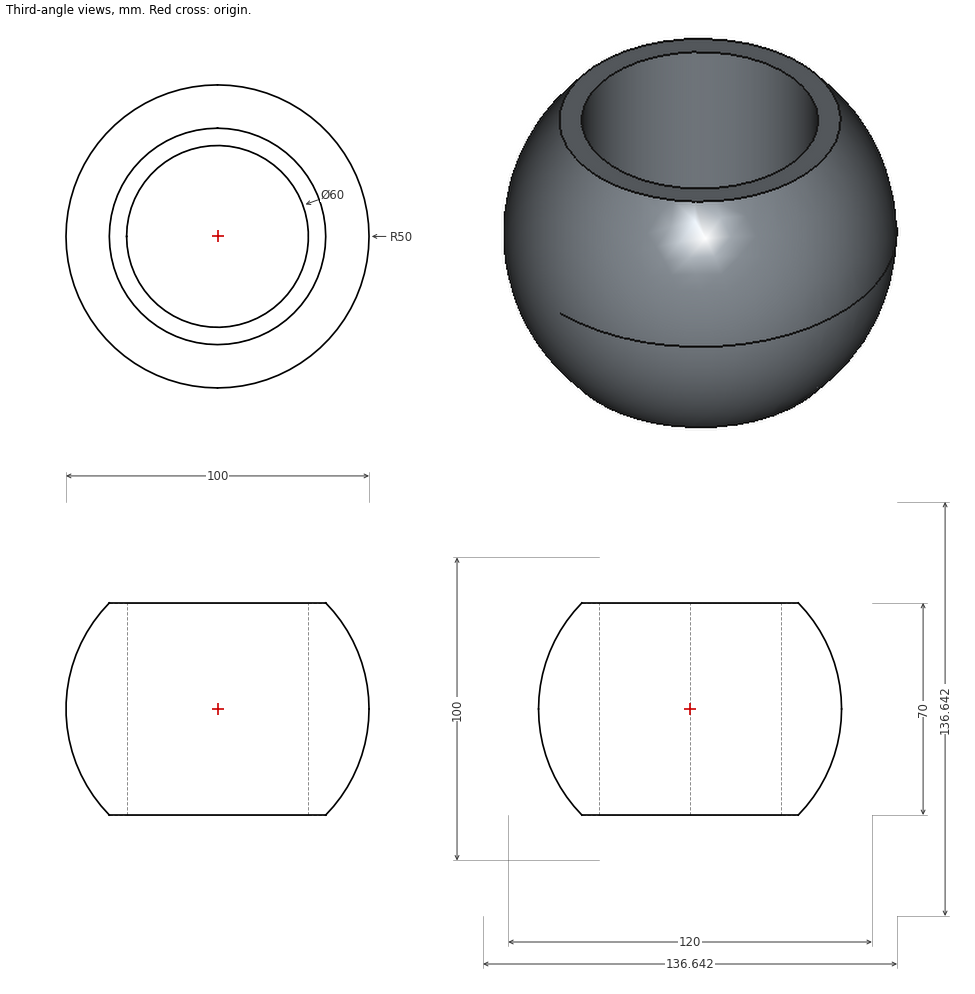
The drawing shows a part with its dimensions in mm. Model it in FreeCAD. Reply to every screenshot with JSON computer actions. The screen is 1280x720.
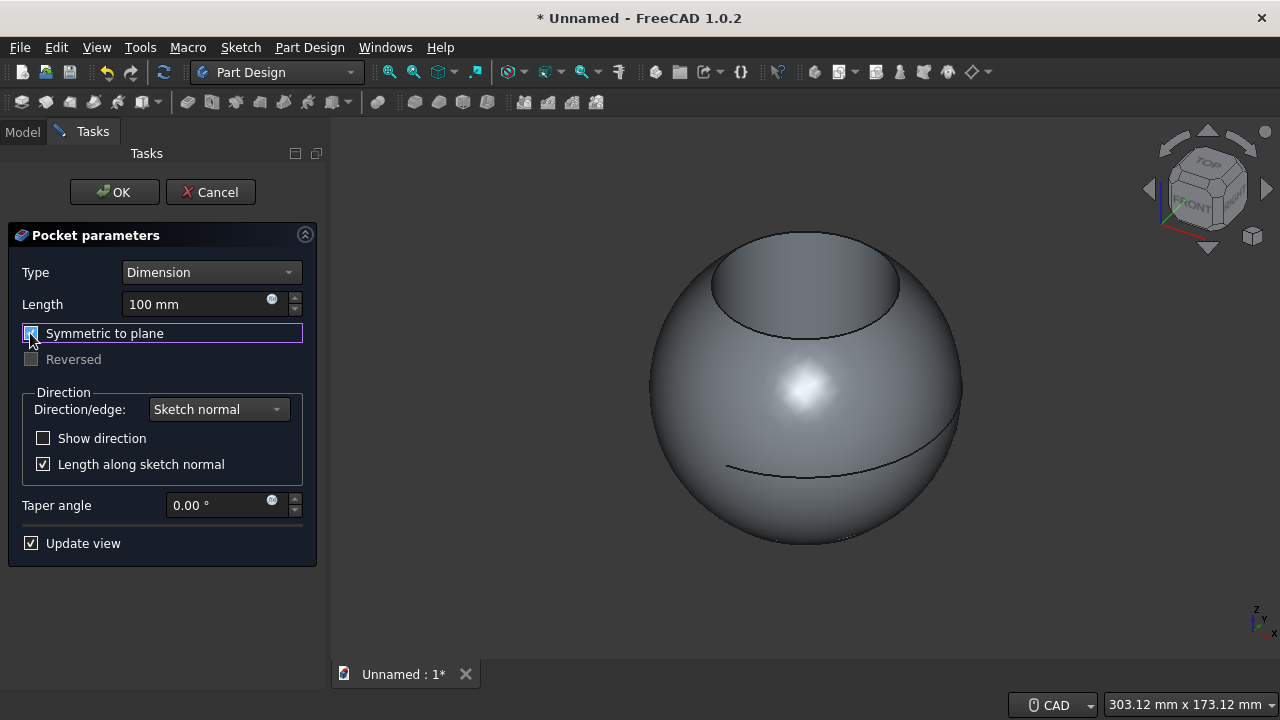
{"action": "left_click", "coordinate": [115, 192]}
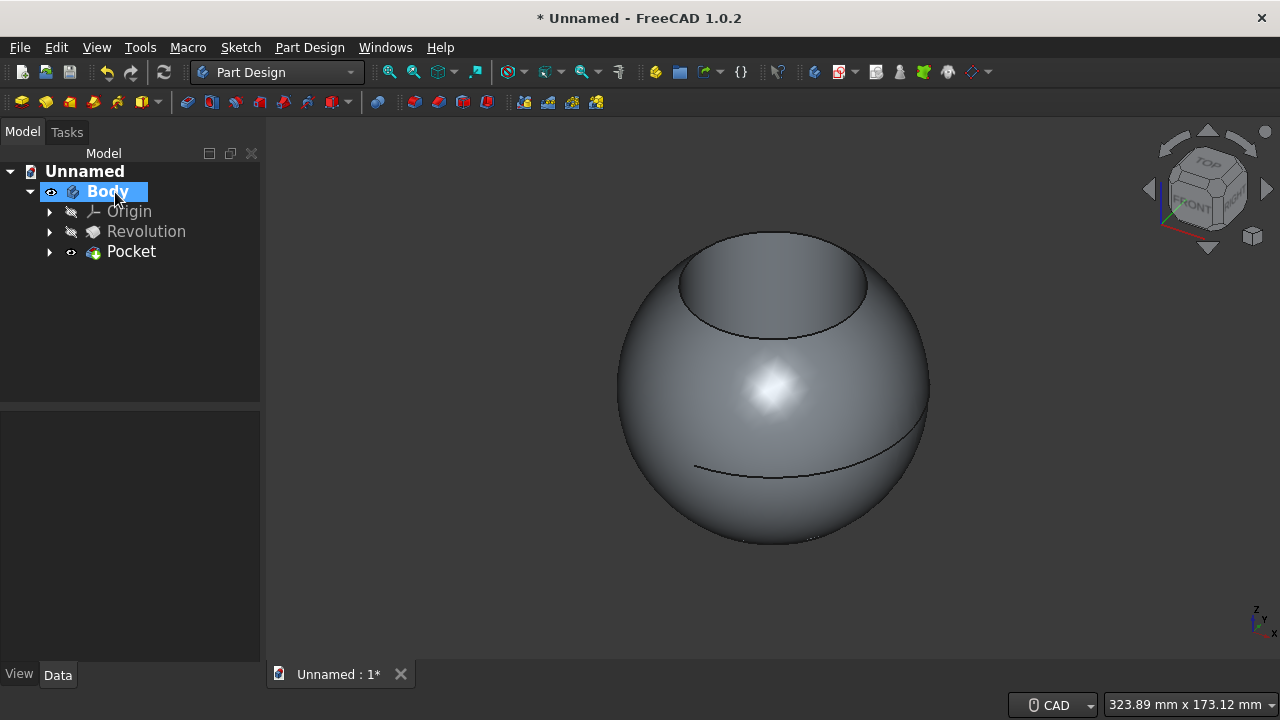
{"action": "left_click", "coordinate": [840, 72]}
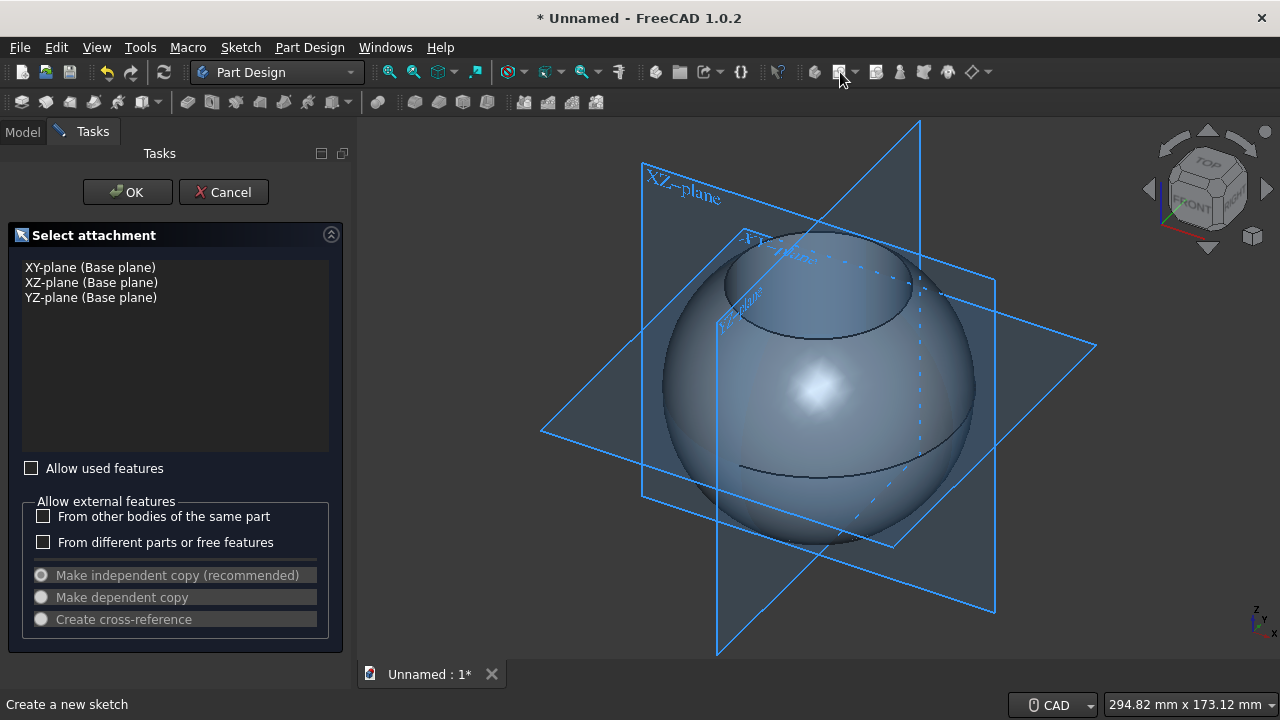
{"action": "left_click", "coordinate": [82, 298]}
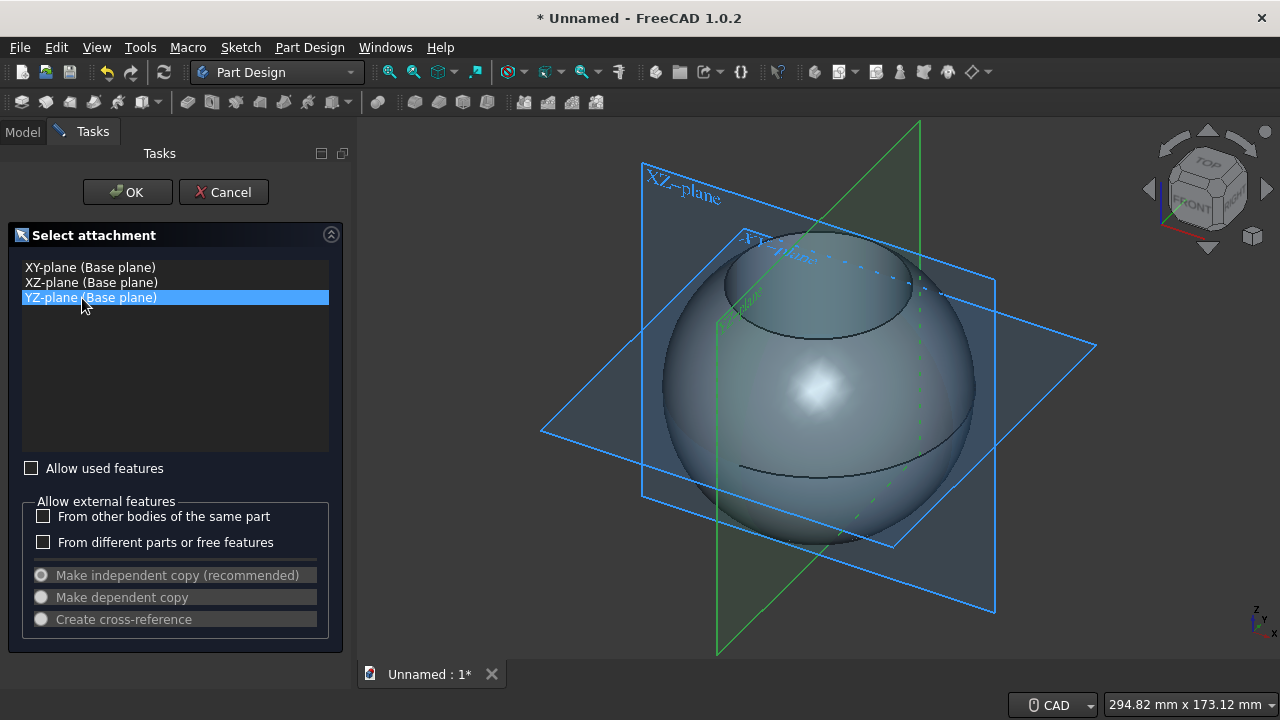
{"action": "left_click", "coordinate": [128, 192]}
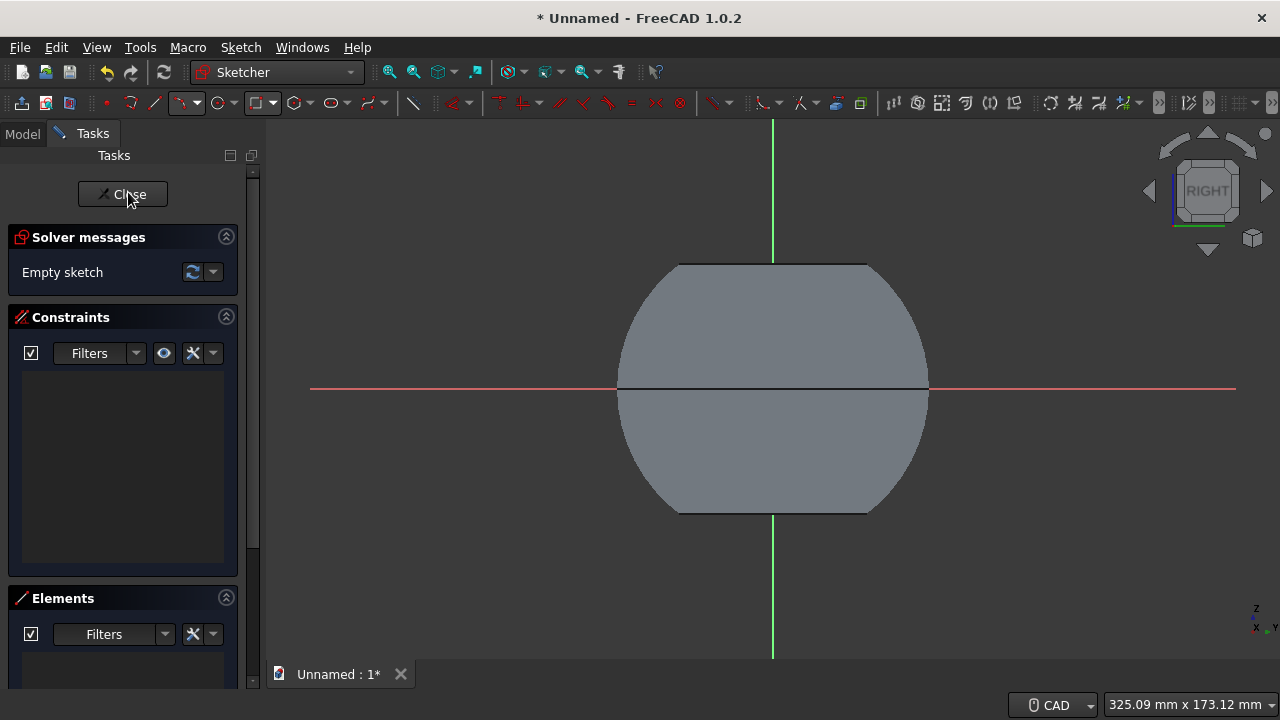
{"action": "left_click", "coordinate": [70, 104]}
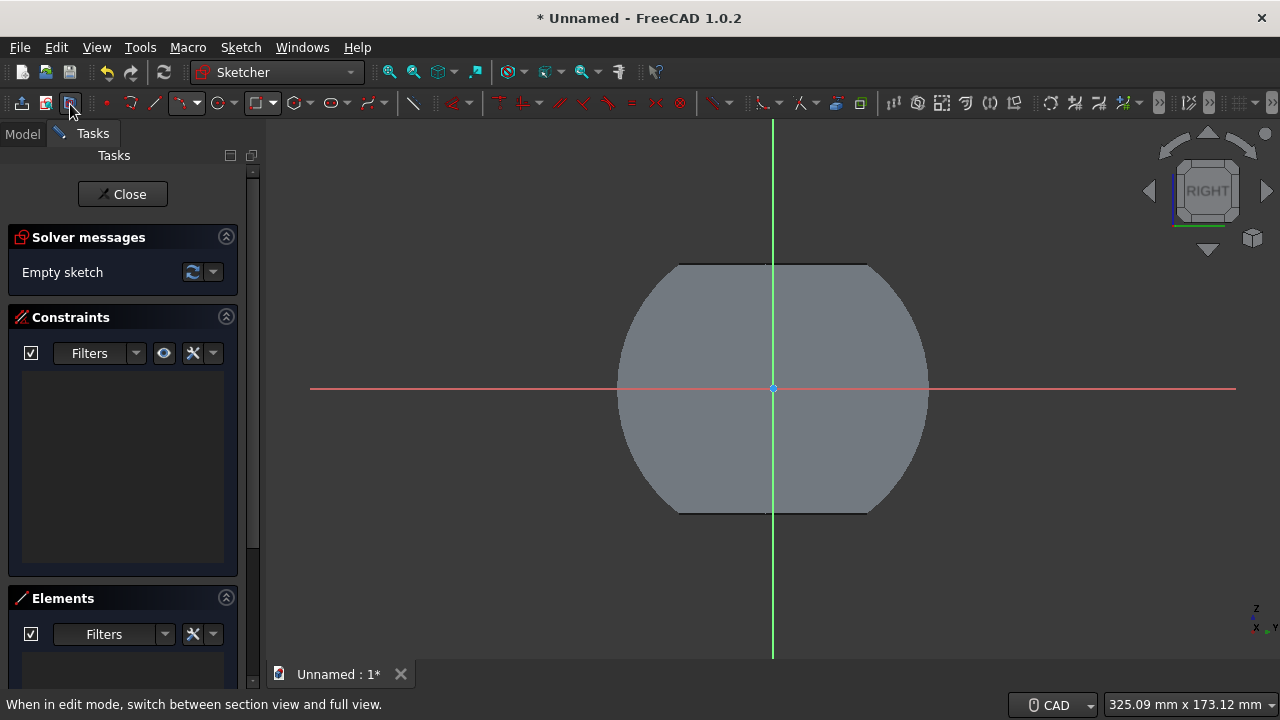
{"action": "key", "text": "g v"}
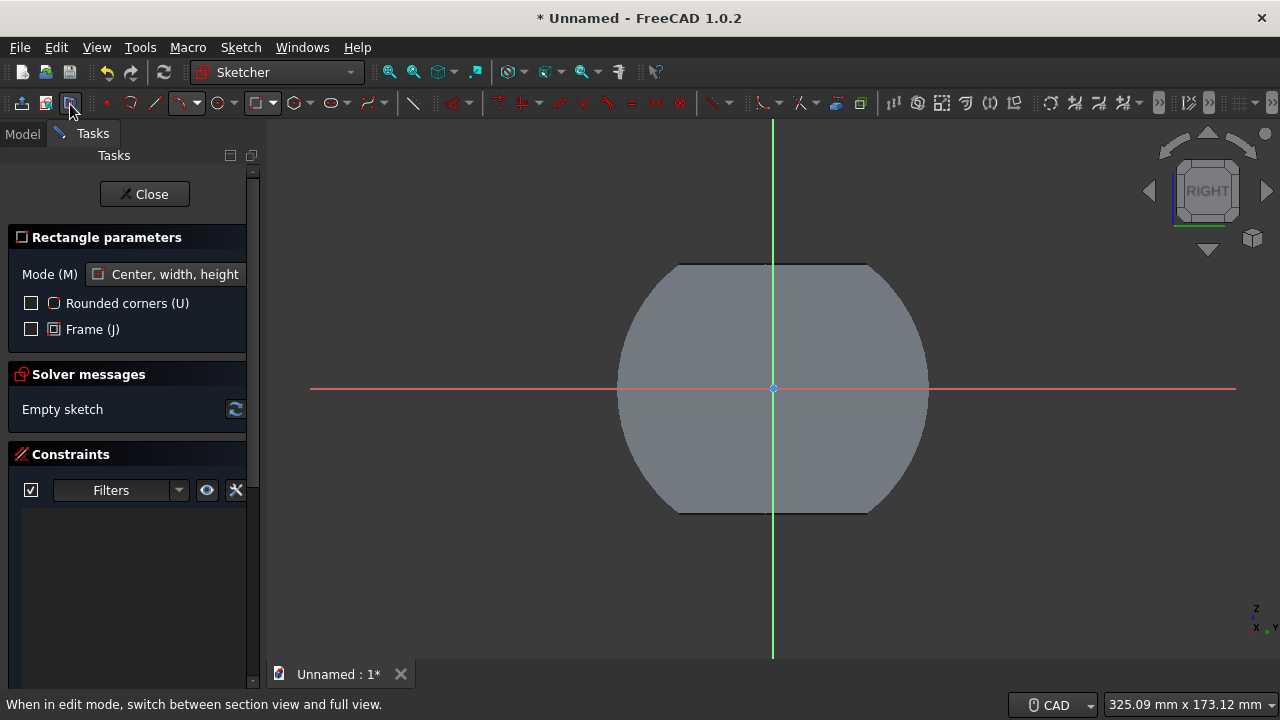
{"action": "left_click", "coordinate": [773, 389]}
{"action": "left_click", "coordinate": [986, 176]}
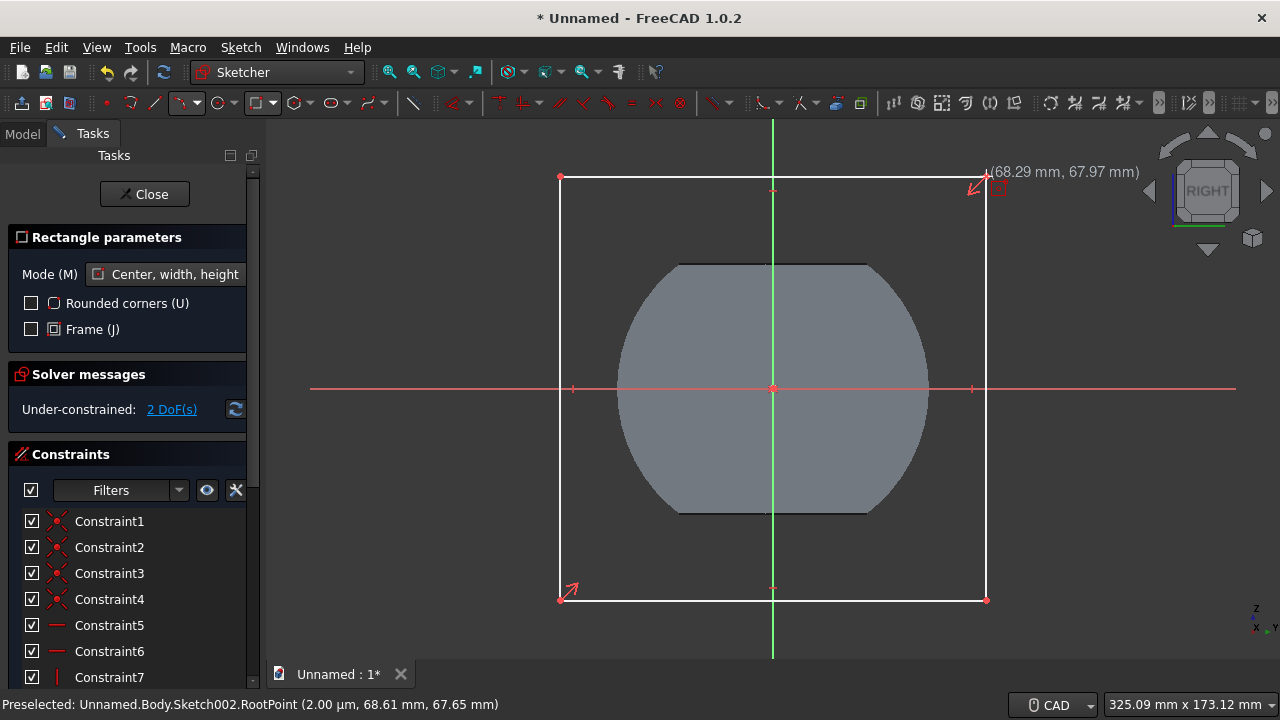
{"action": "left_click", "coordinate": [773, 389]}
{"action": "left_click", "coordinate": [960, 280]}
{"action": "key", "text": "Escape"}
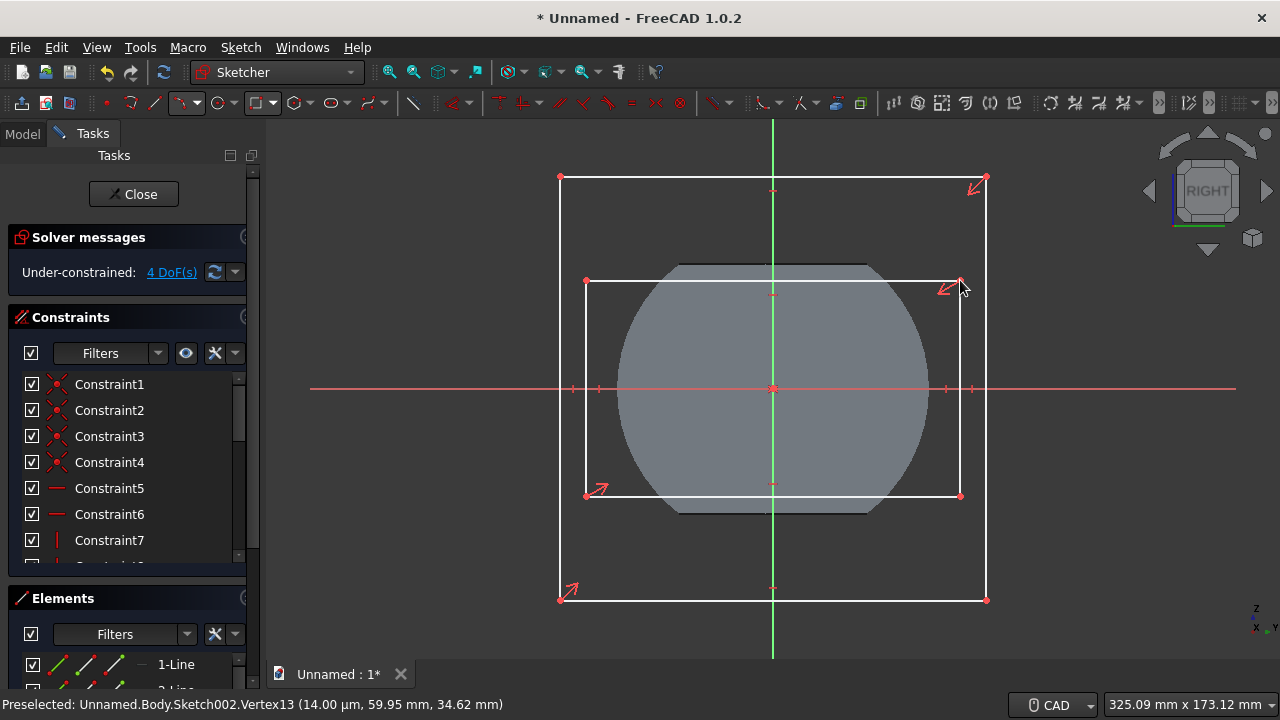
{"action": "left_click", "coordinate": [452, 104]}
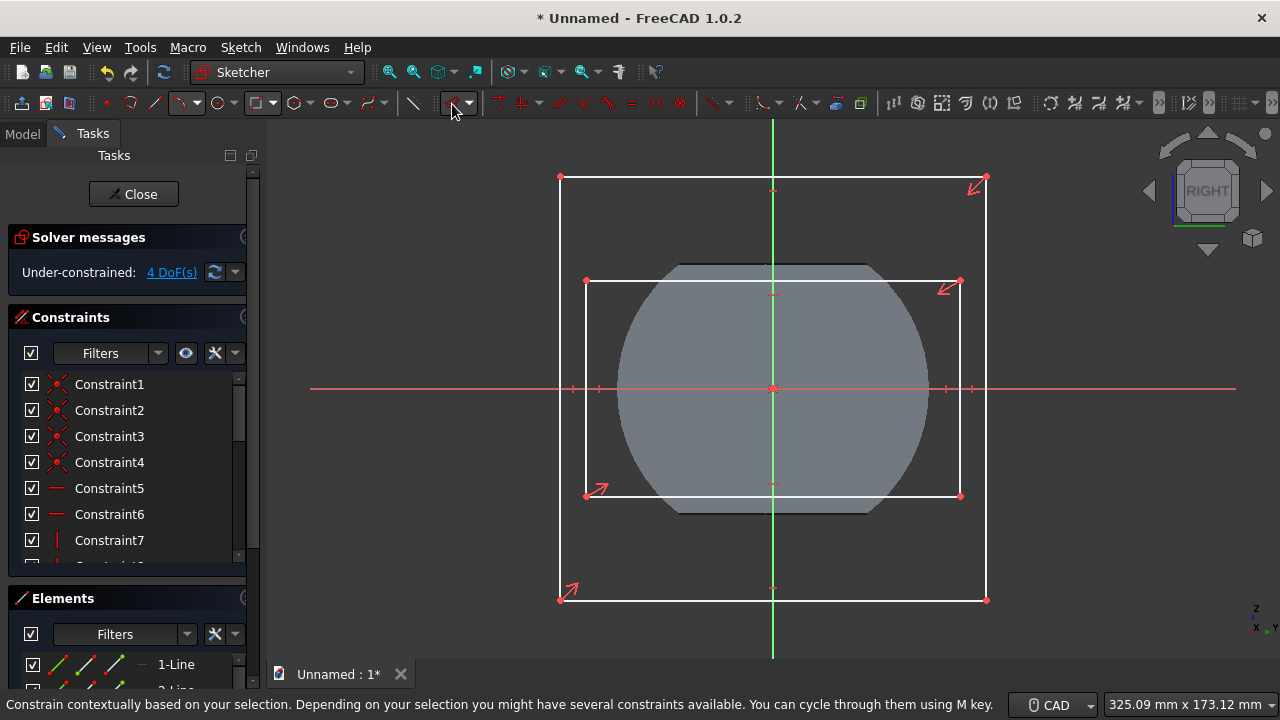
{"action": "left_click", "coordinate": [960, 432]}
{"action": "left_click", "coordinate": [926, 339]}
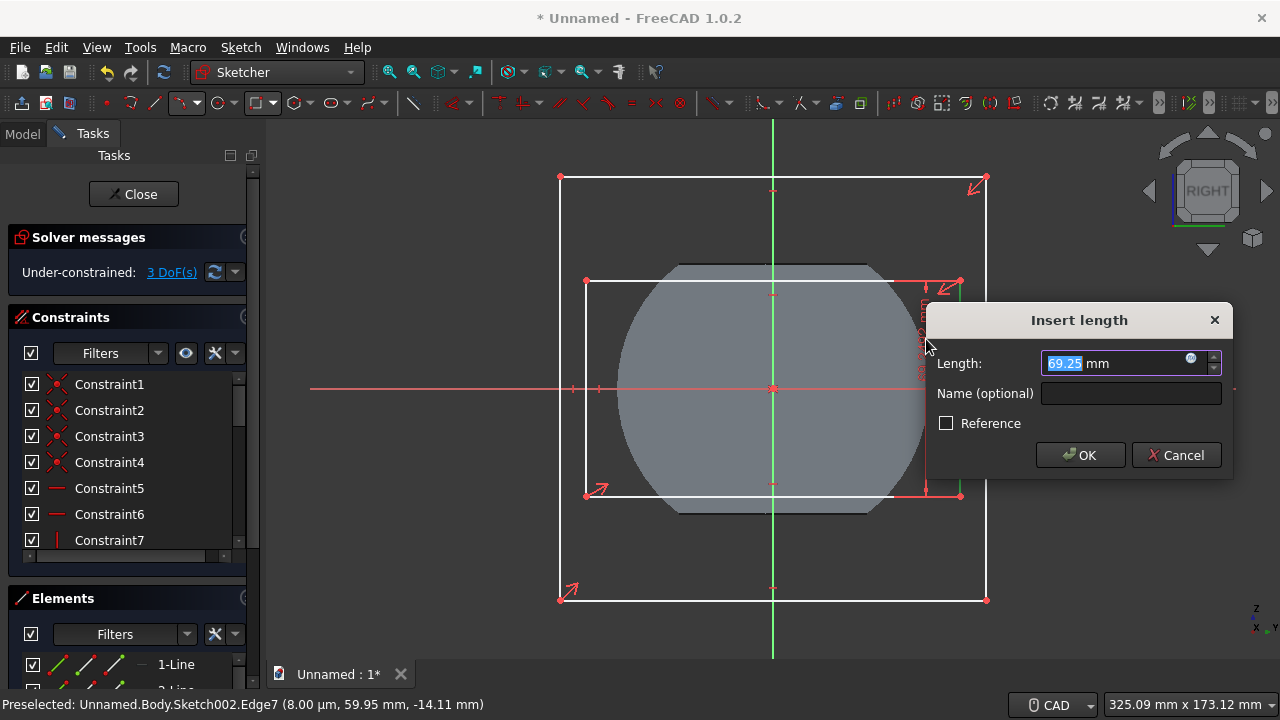
{"action": "type", "text": "70"}
{"action": "key", "text": "Return"}